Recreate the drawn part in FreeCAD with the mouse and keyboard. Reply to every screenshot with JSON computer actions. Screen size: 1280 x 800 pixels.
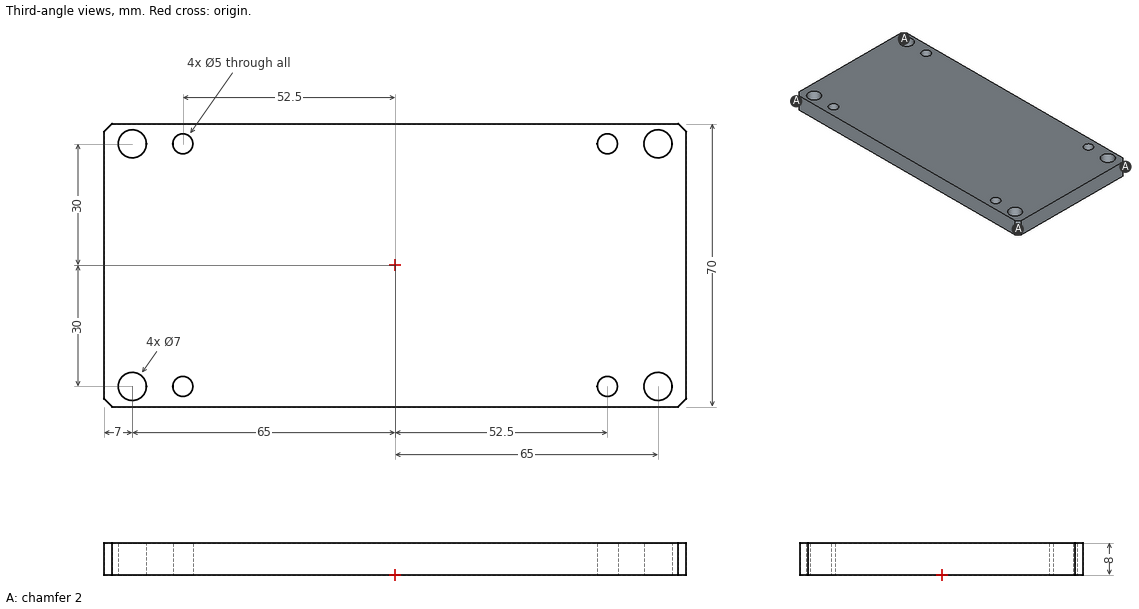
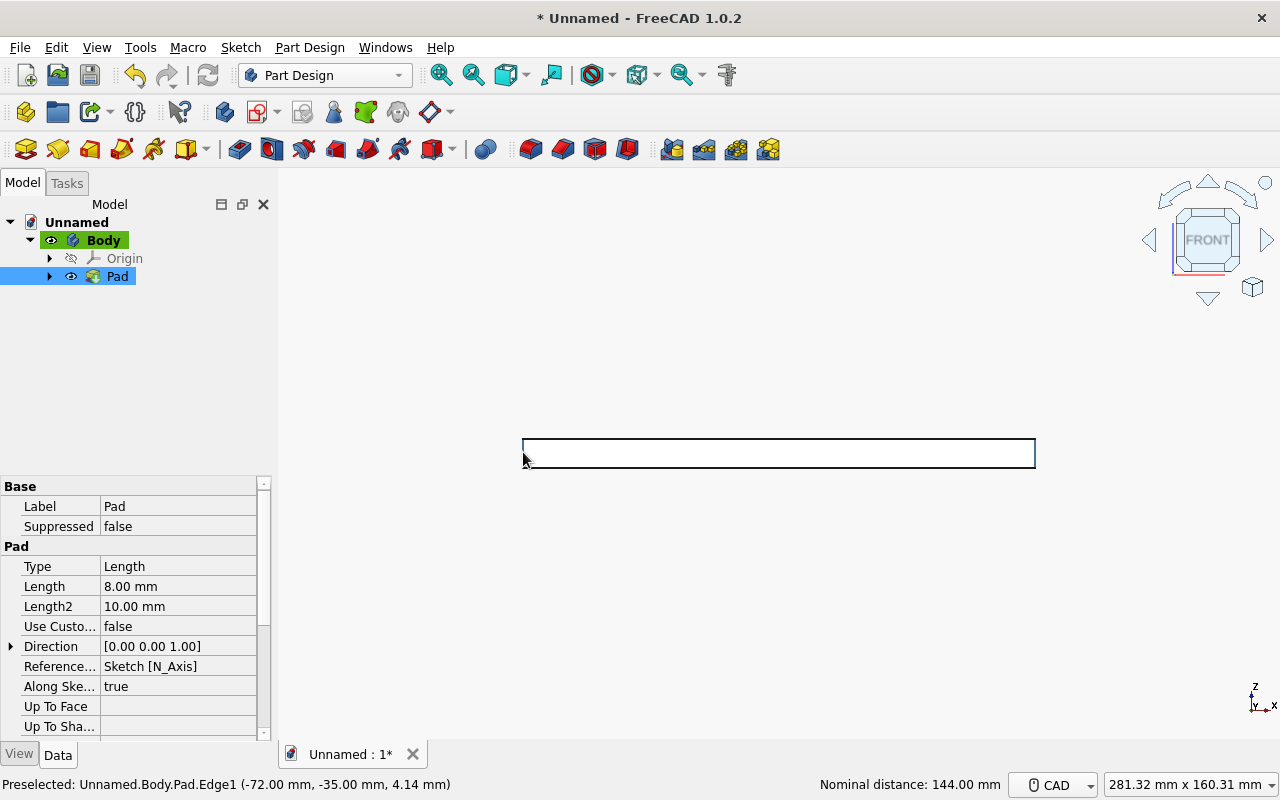
{"action": "key", "text": "3"}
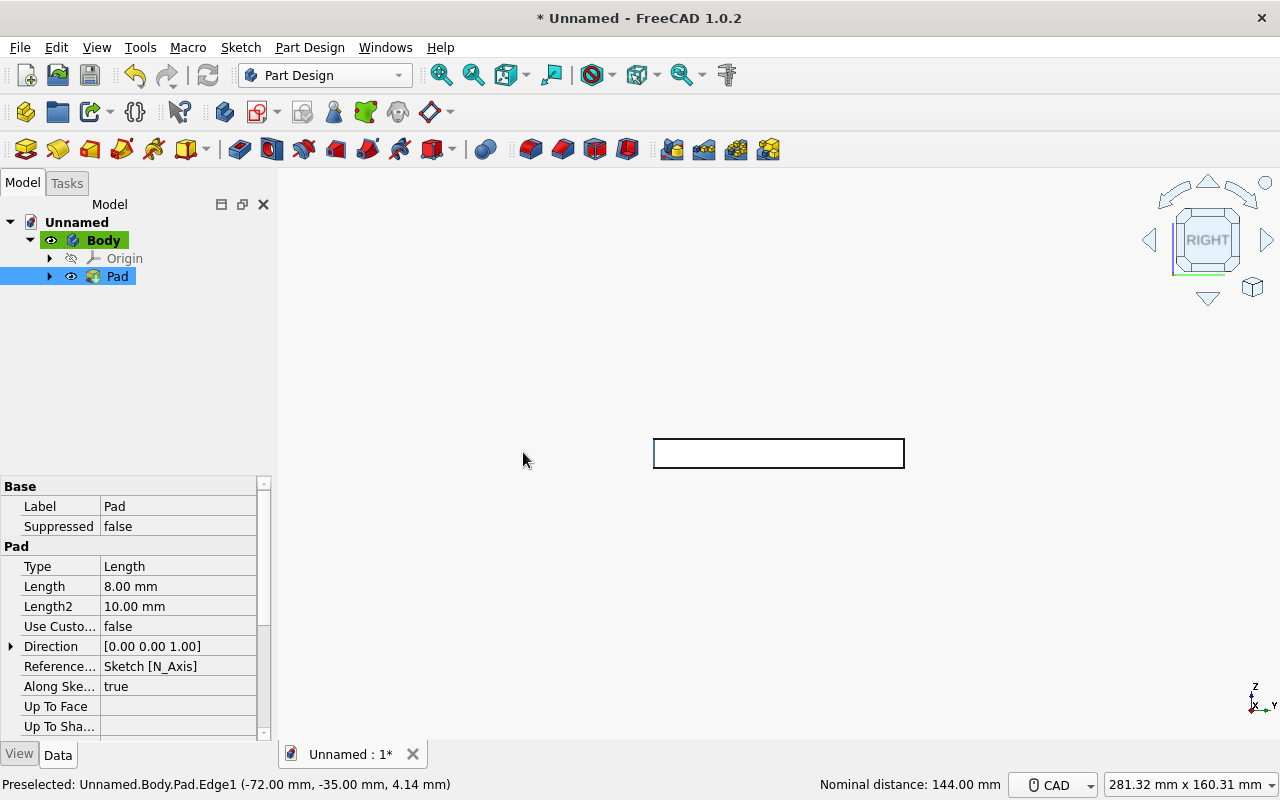
{"action": "left_click", "coordinate": [442, 76]}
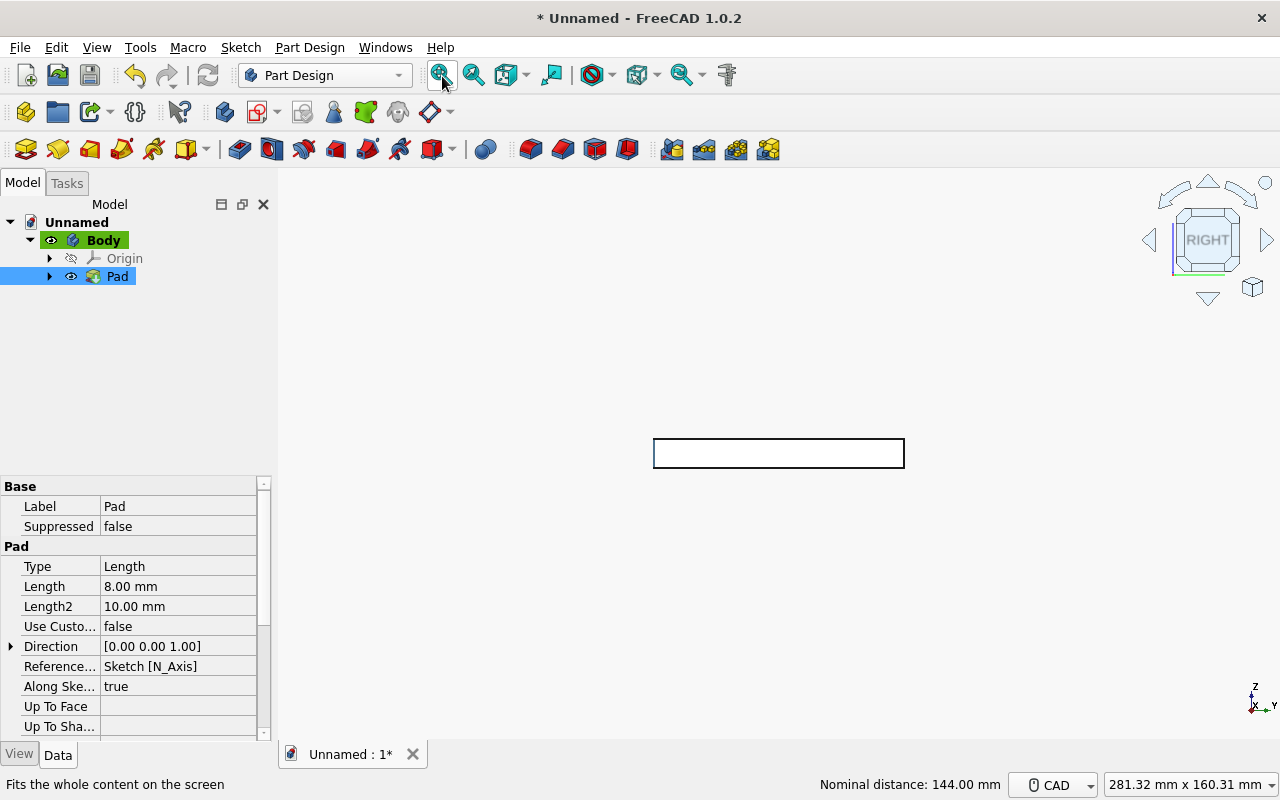
{"action": "left_click", "coordinate": [904, 452], "text": "ctrl"}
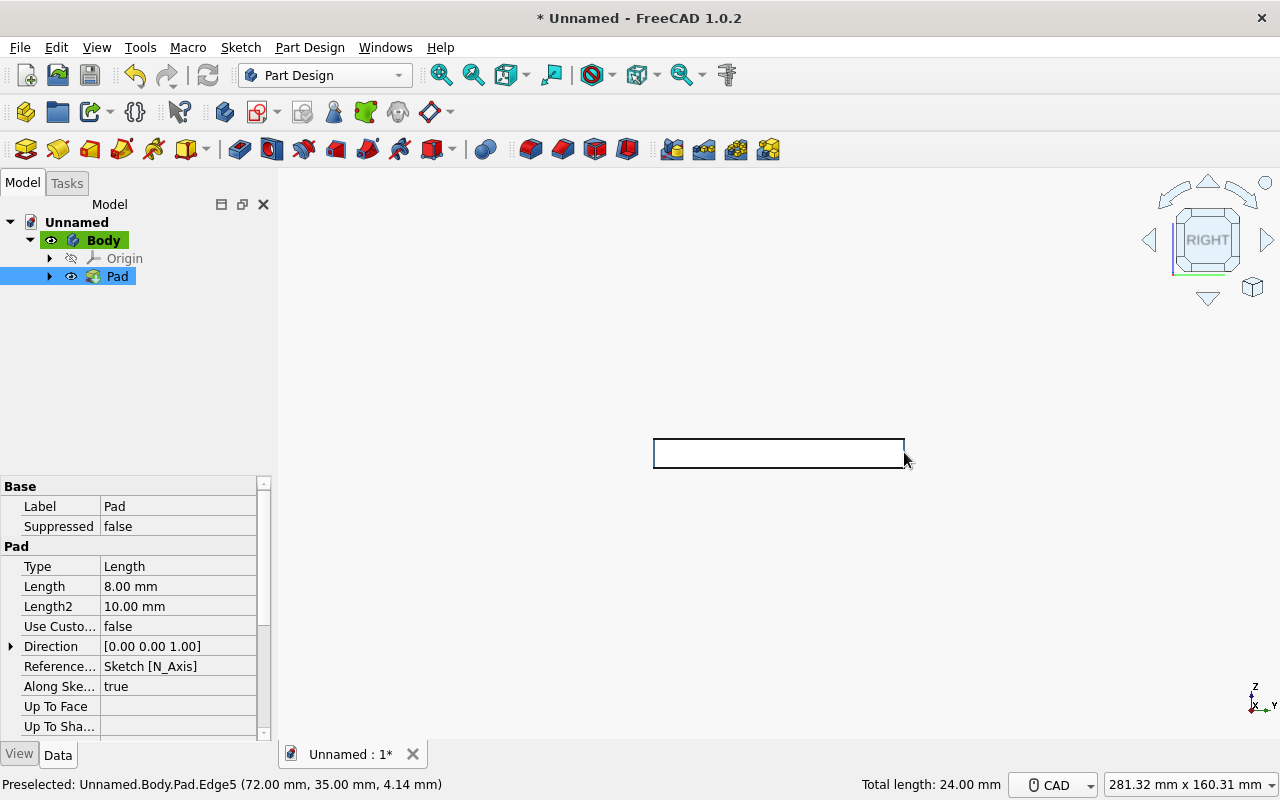
{"action": "key", "text": "5"}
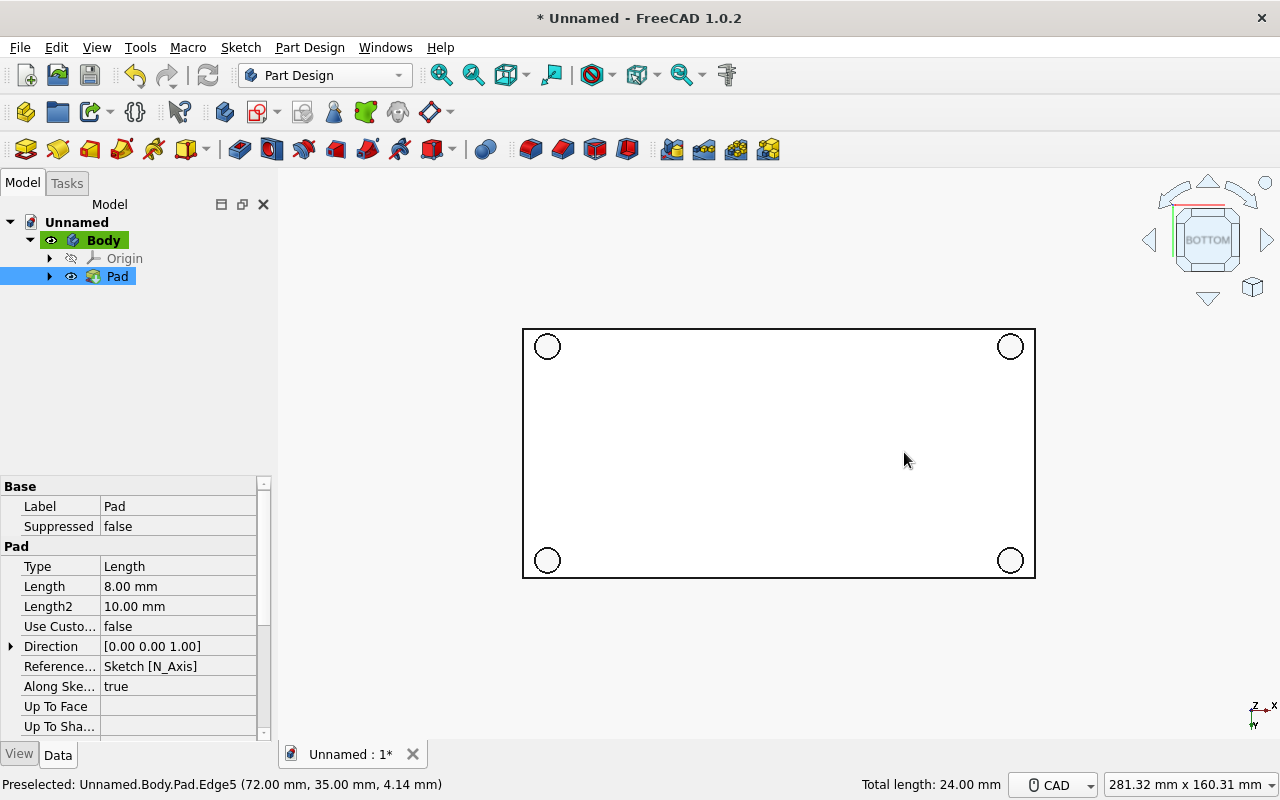
{"action": "key", "text": "4"}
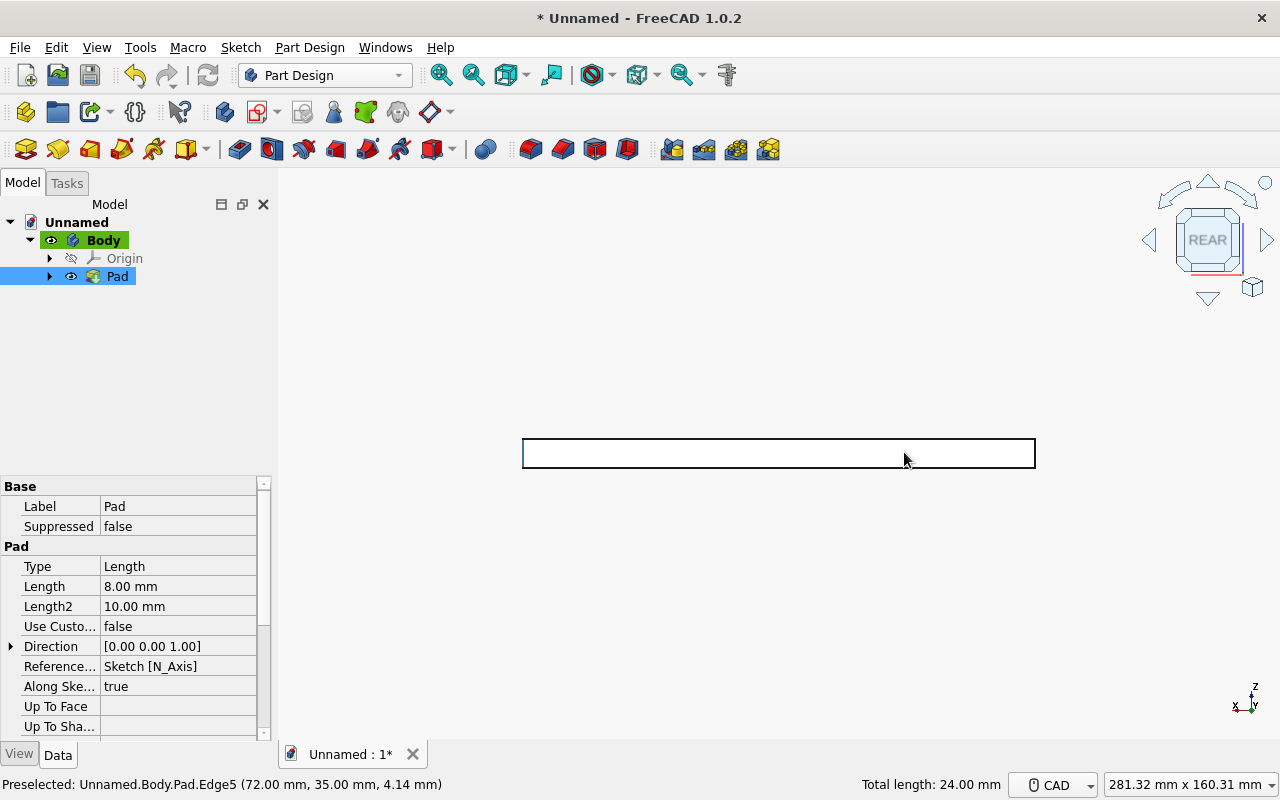
{"action": "left_click", "coordinate": [1035, 452], "text": "ctrl"}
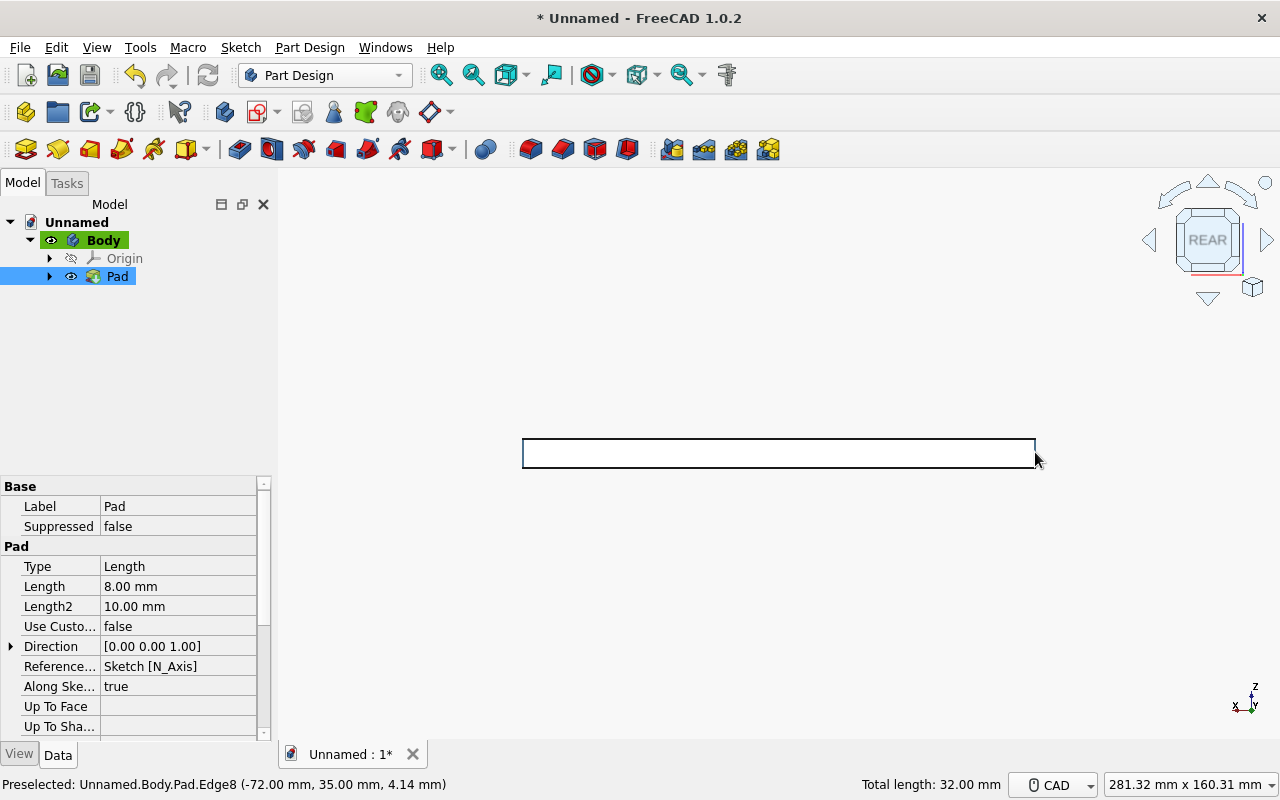
{"action": "left_click", "coordinate": [564, 150]}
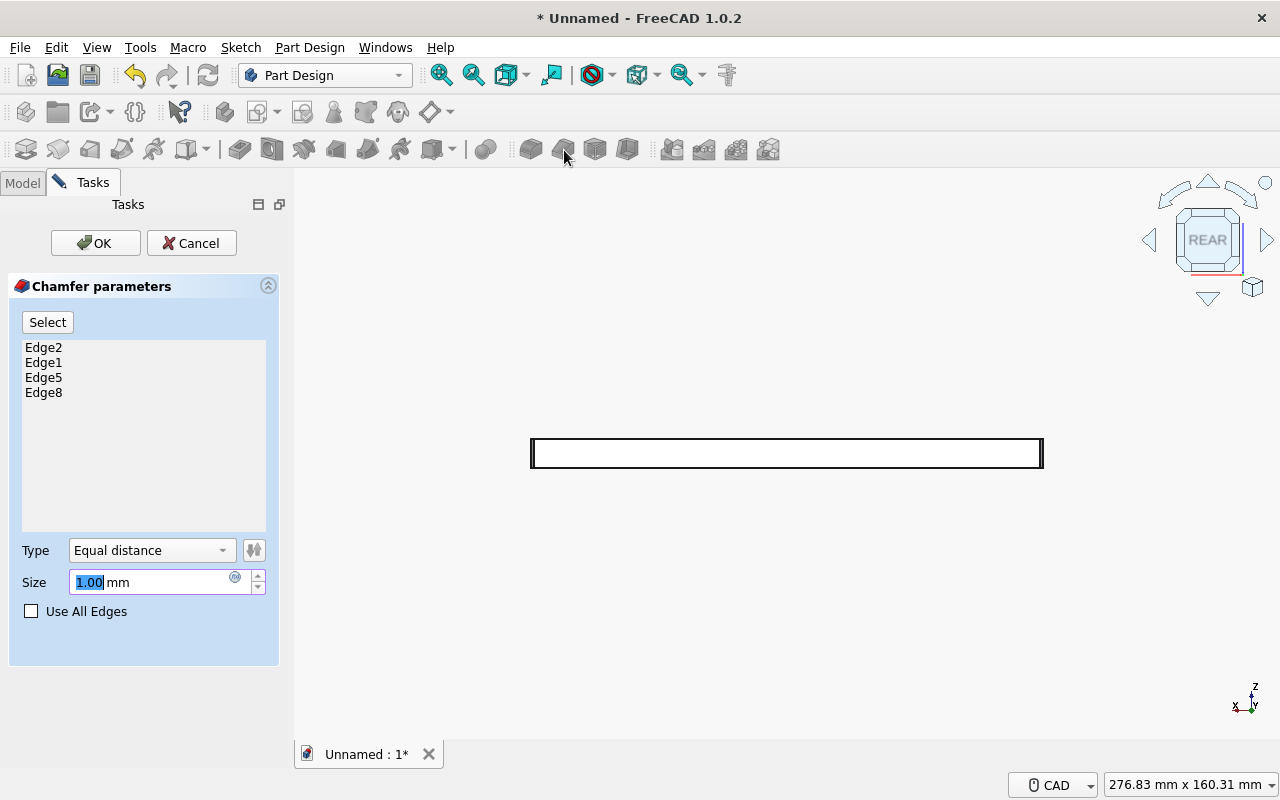
{"action": "type", "text": "2"}
{"action": "key", "text": "Tab"}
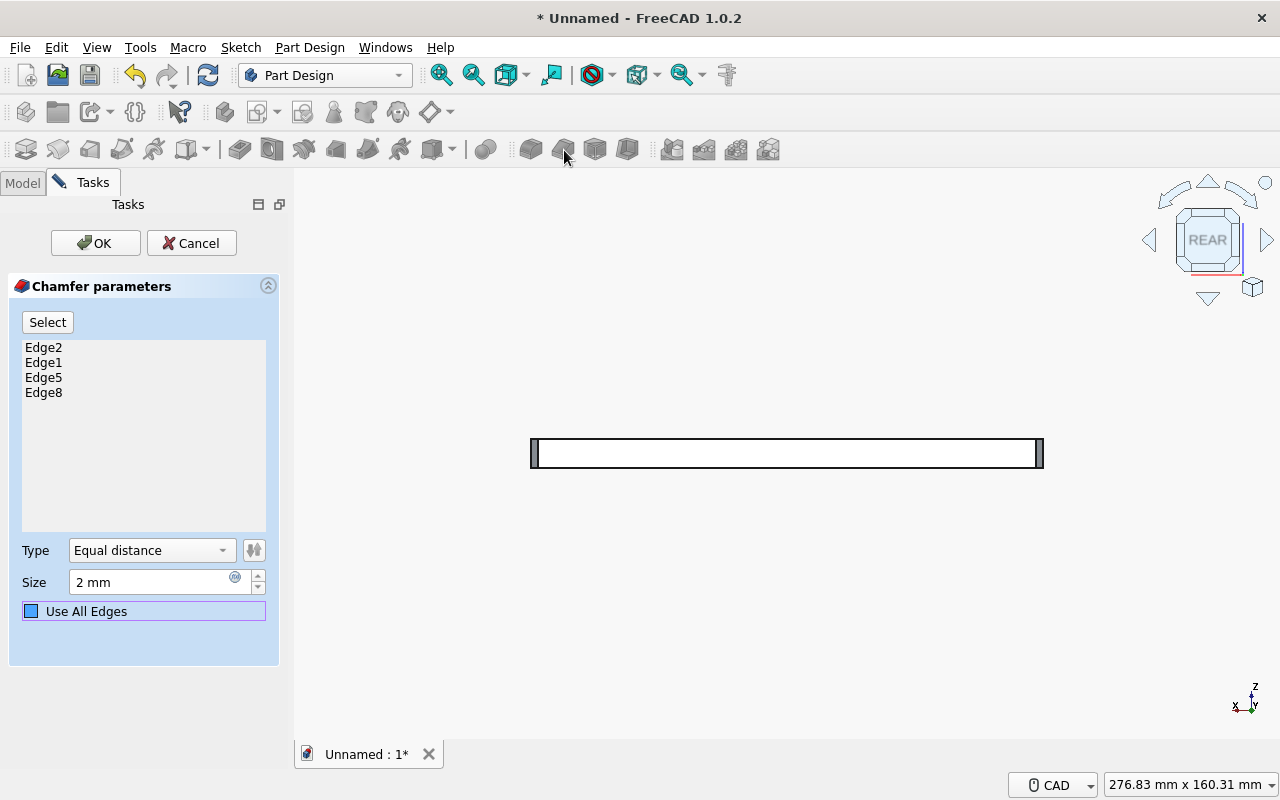
{"action": "left_click", "coordinate": [96, 243]}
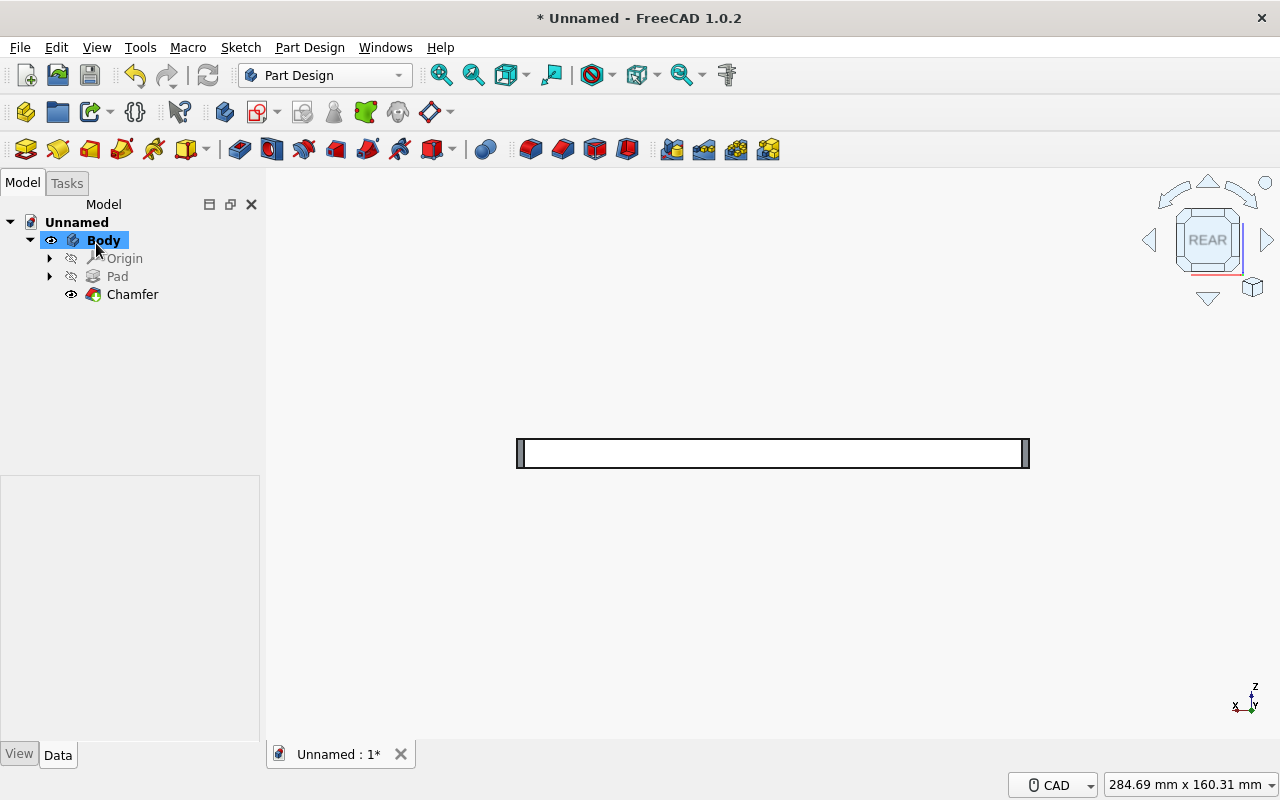
{"action": "key", "text": "0"}